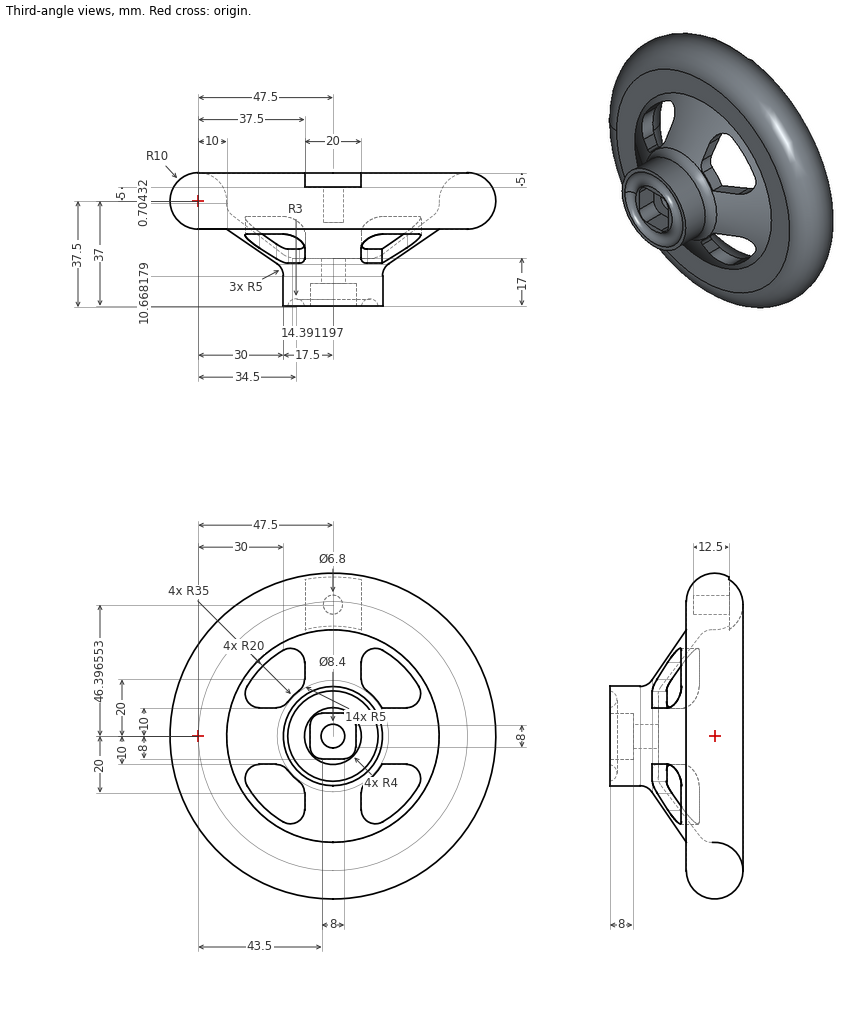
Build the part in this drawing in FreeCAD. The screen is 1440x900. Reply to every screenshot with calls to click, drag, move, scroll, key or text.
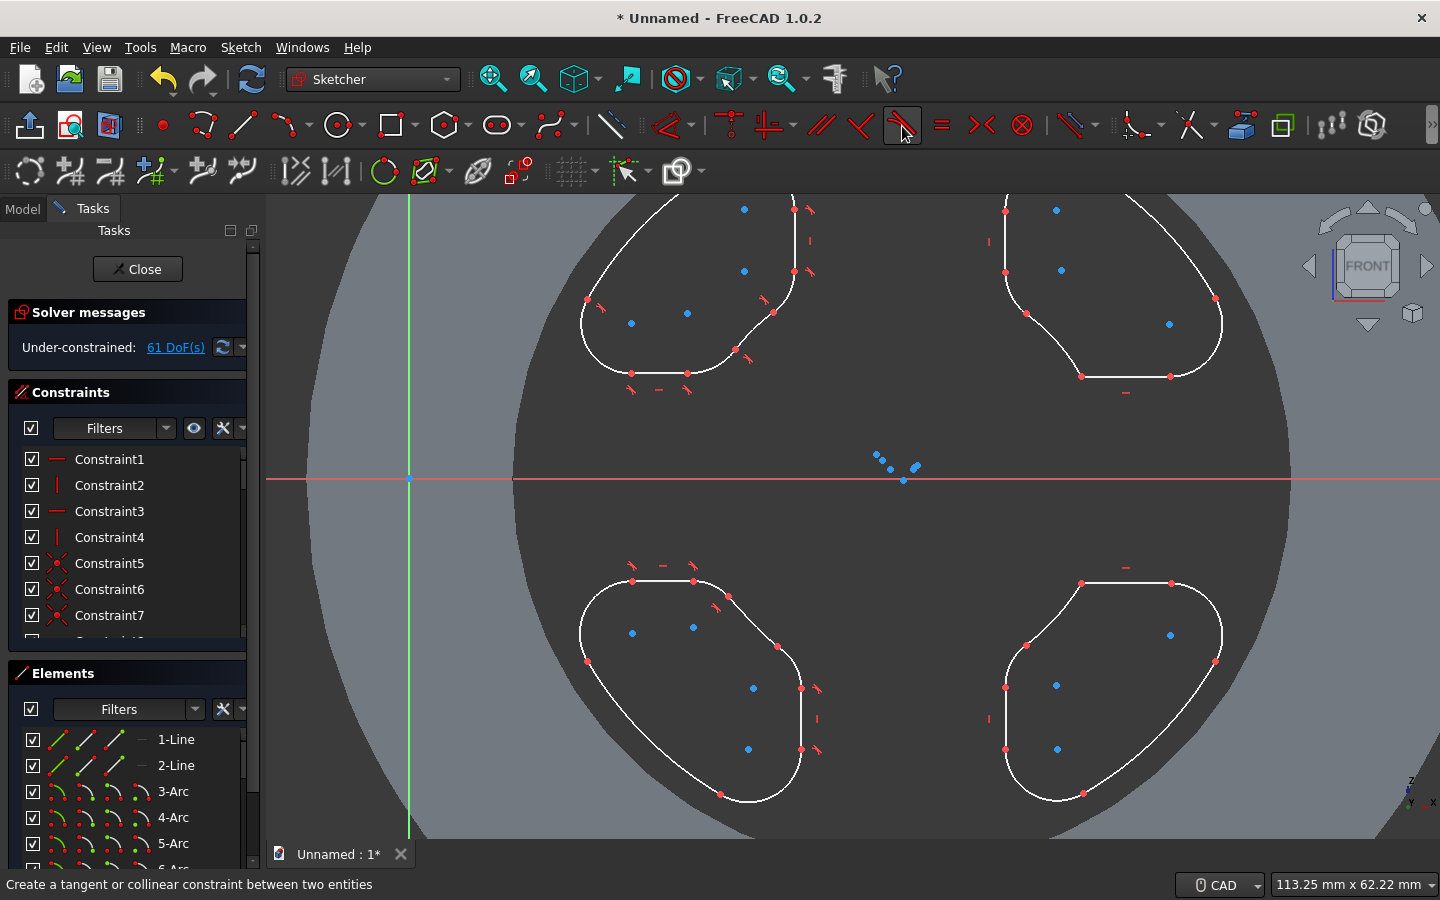
click(743, 612)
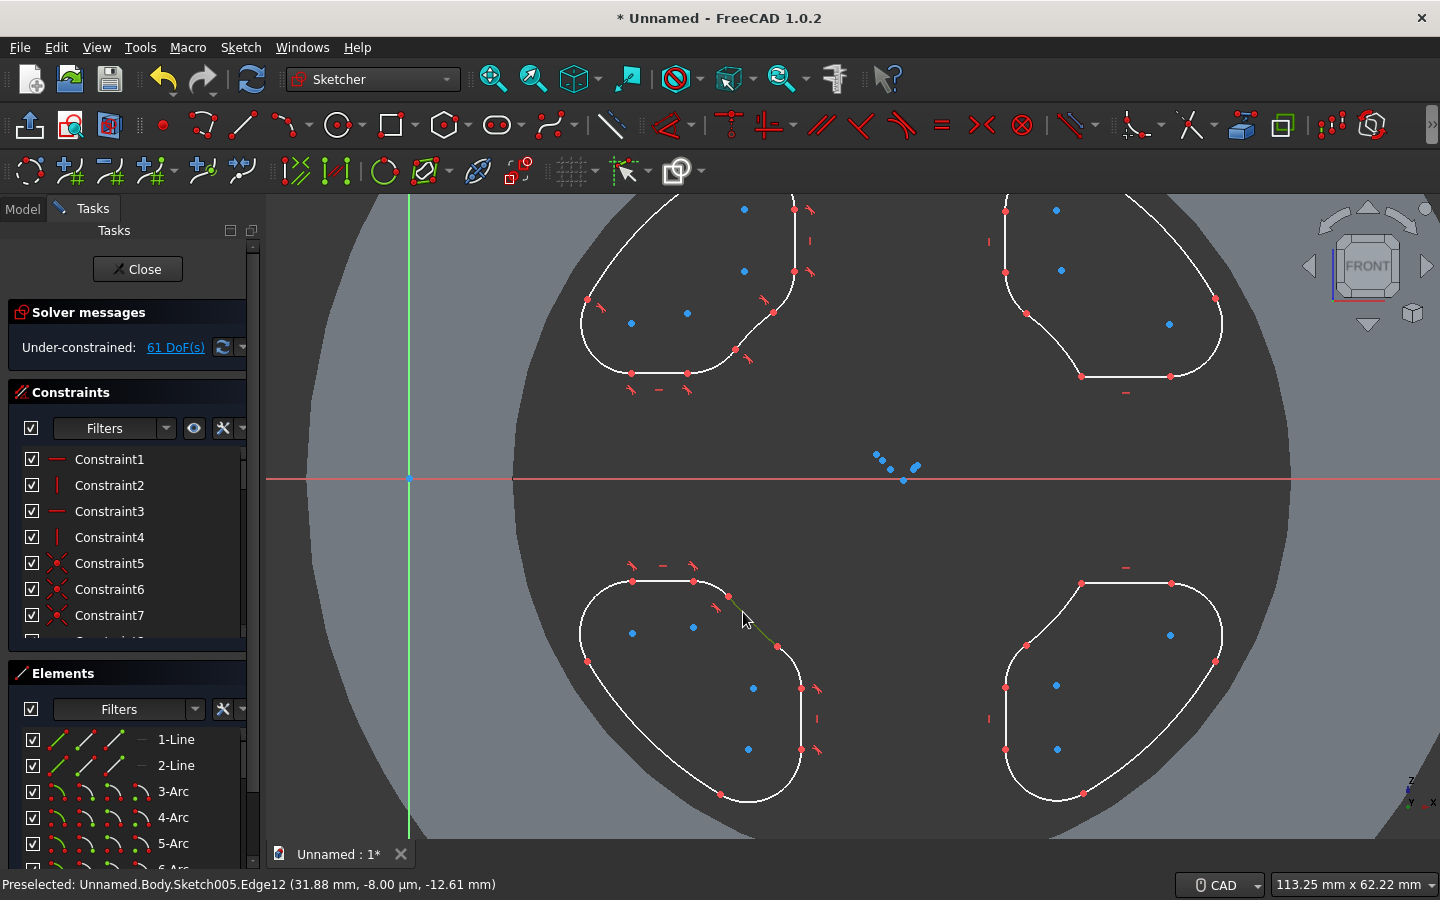
click(799, 673)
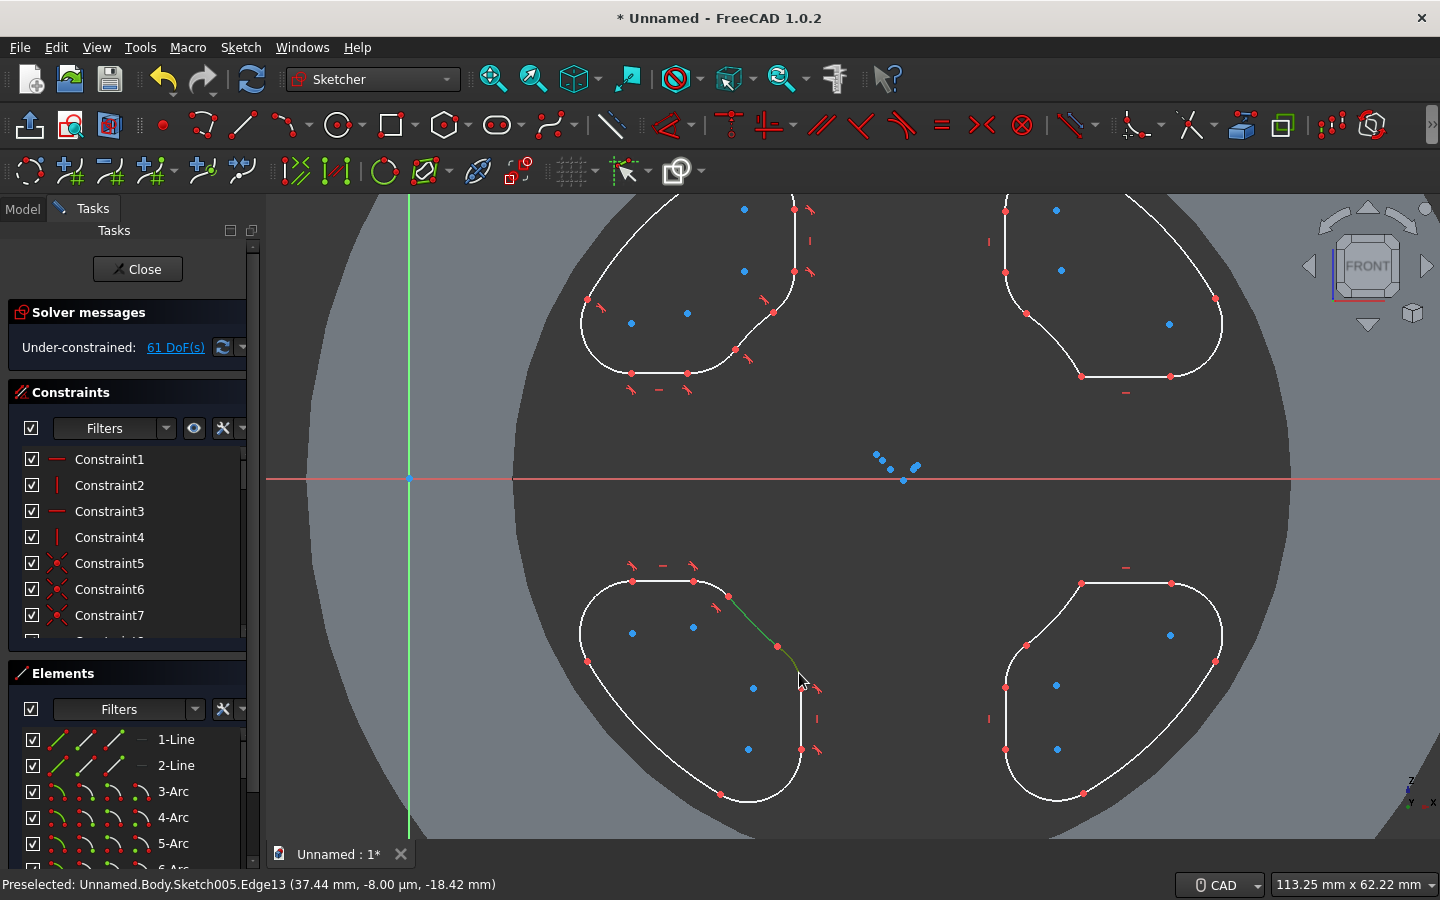
click(902, 126)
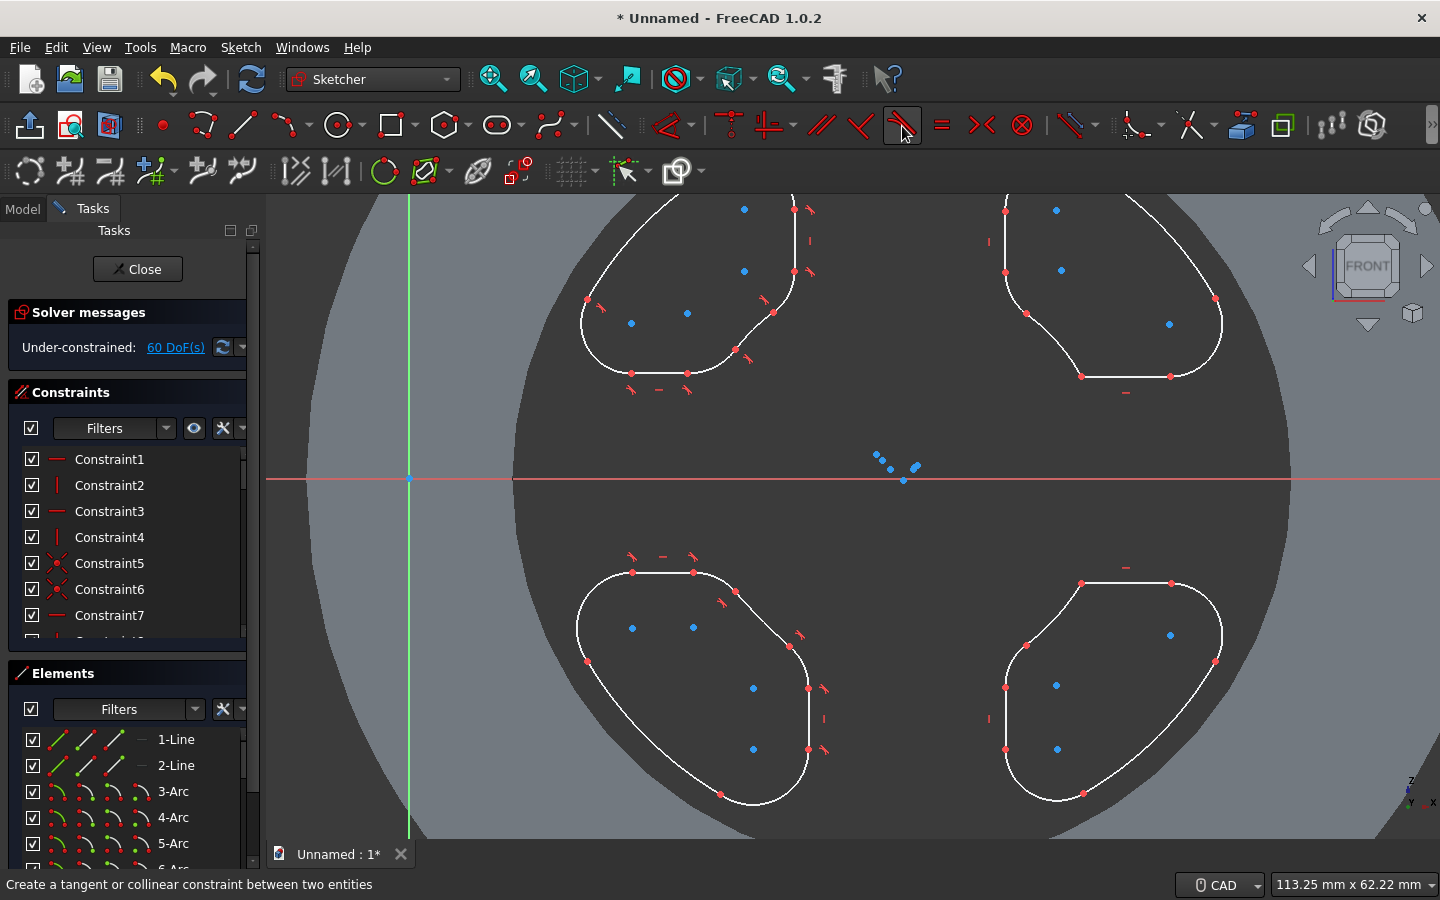
click(755, 805)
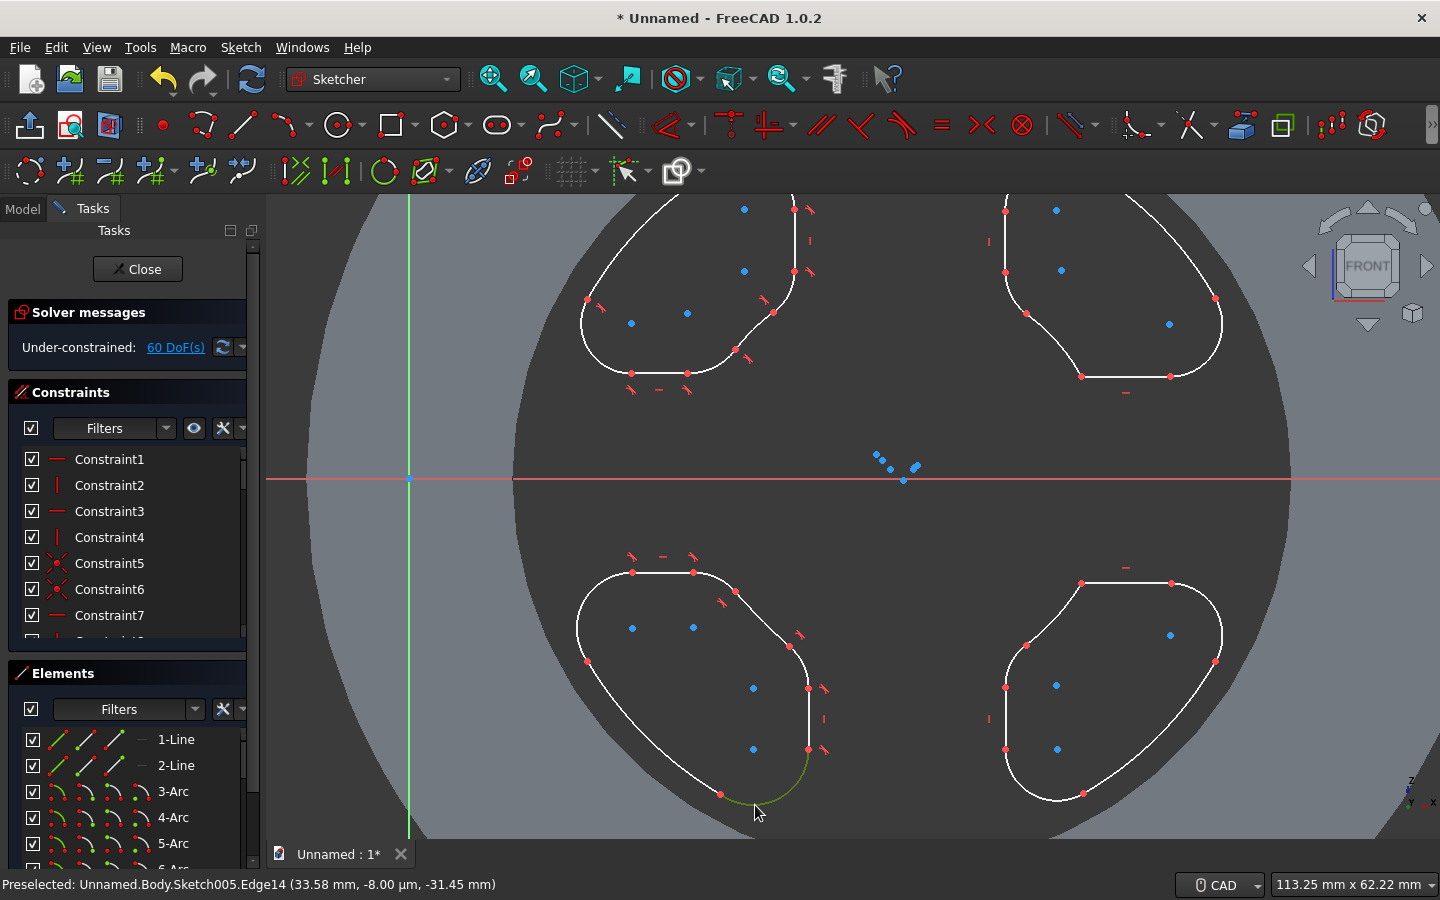
click(620, 708)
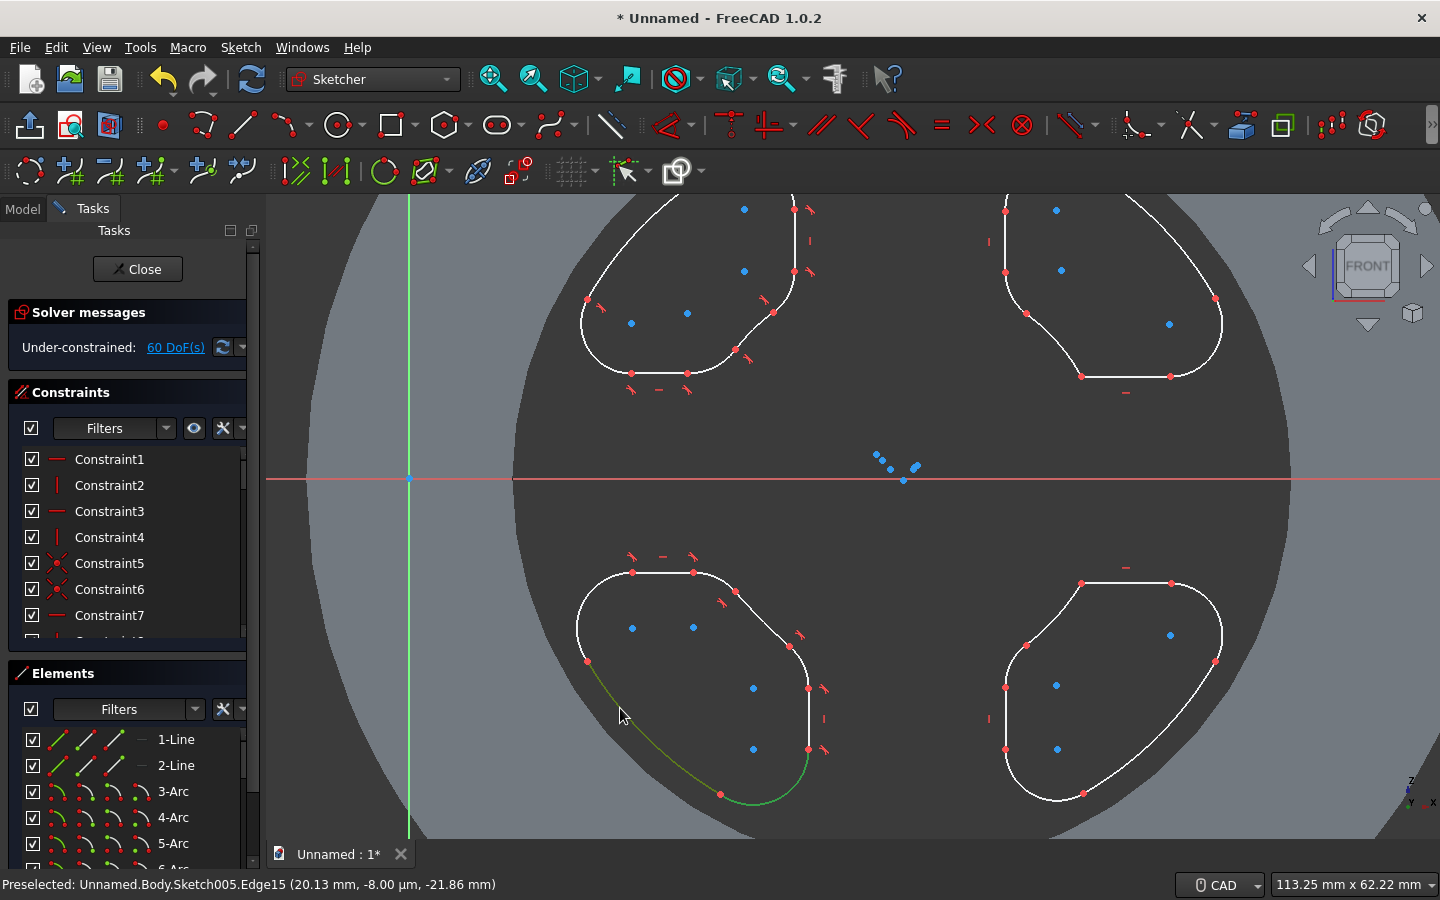
click(902, 126)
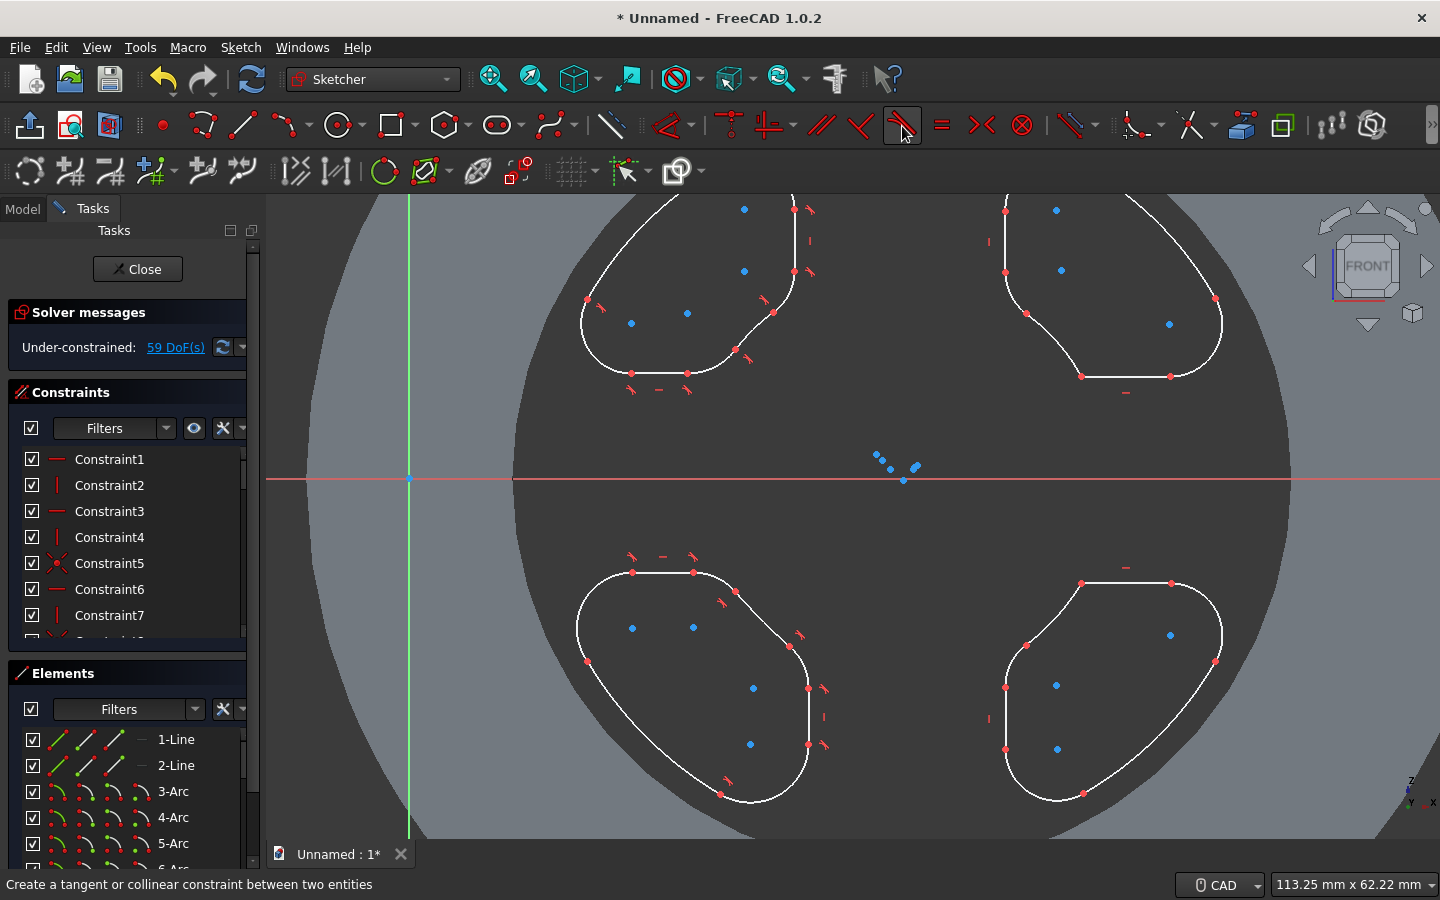
click(620, 708)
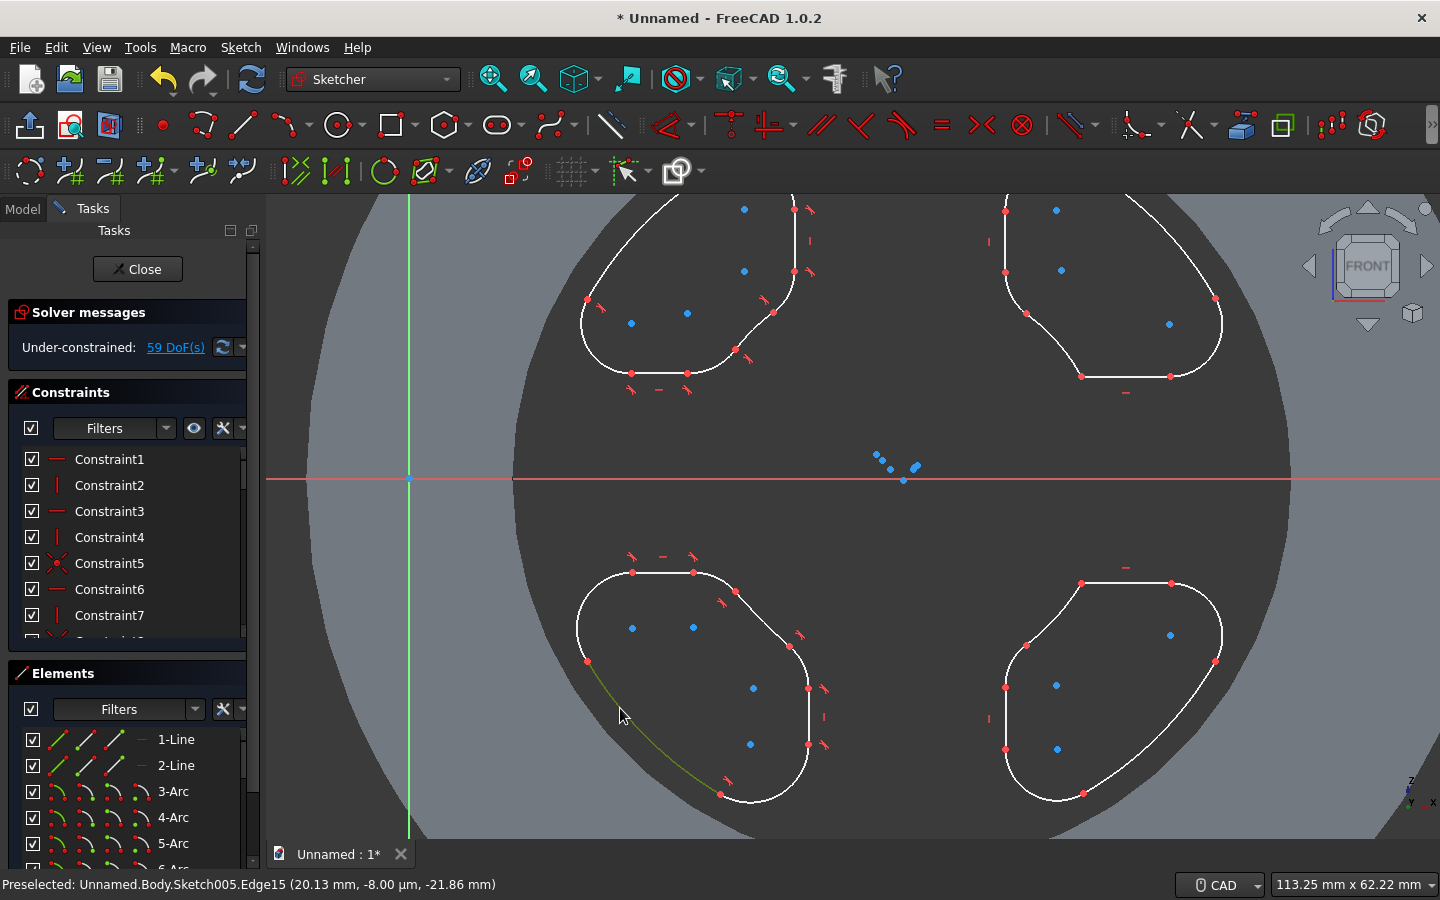
click(598, 585)